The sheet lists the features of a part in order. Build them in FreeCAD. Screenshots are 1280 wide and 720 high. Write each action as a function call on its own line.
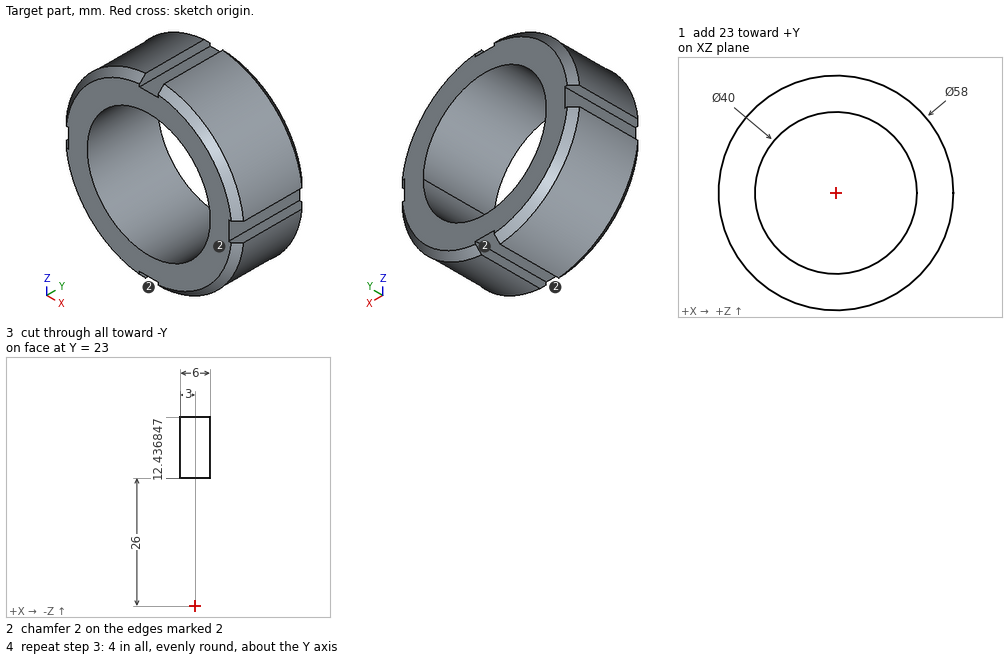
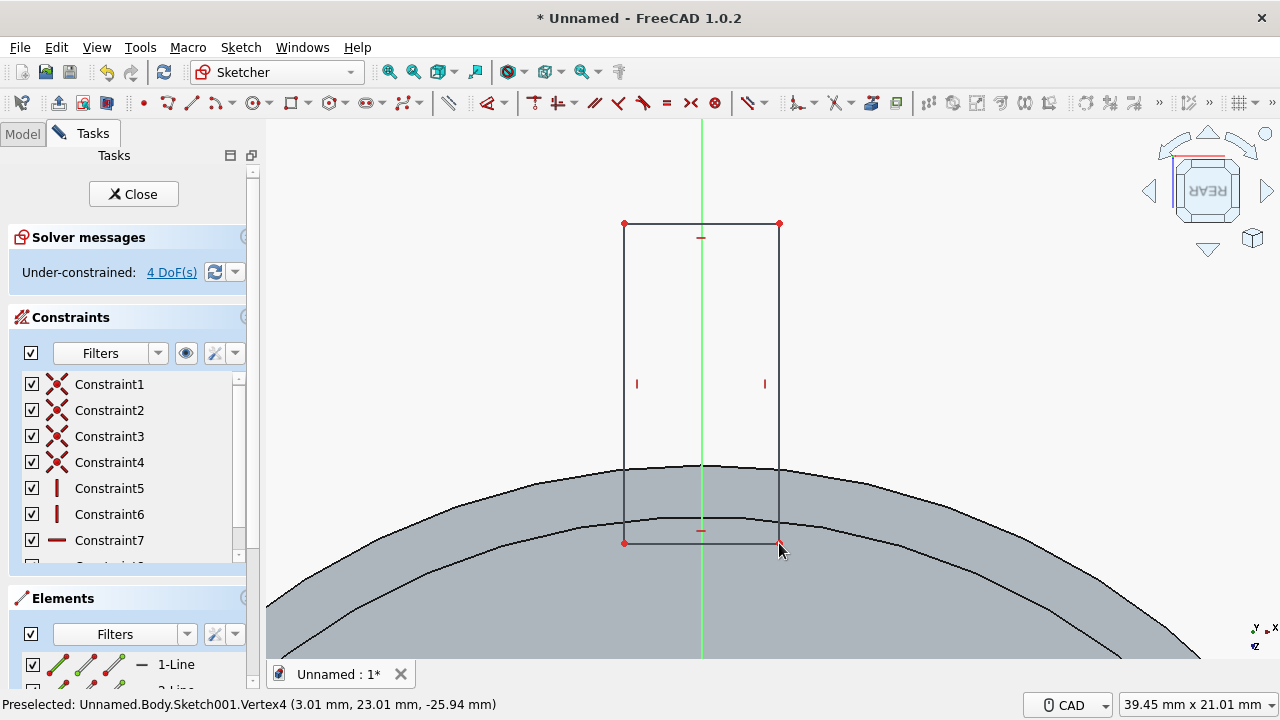
click(488, 104)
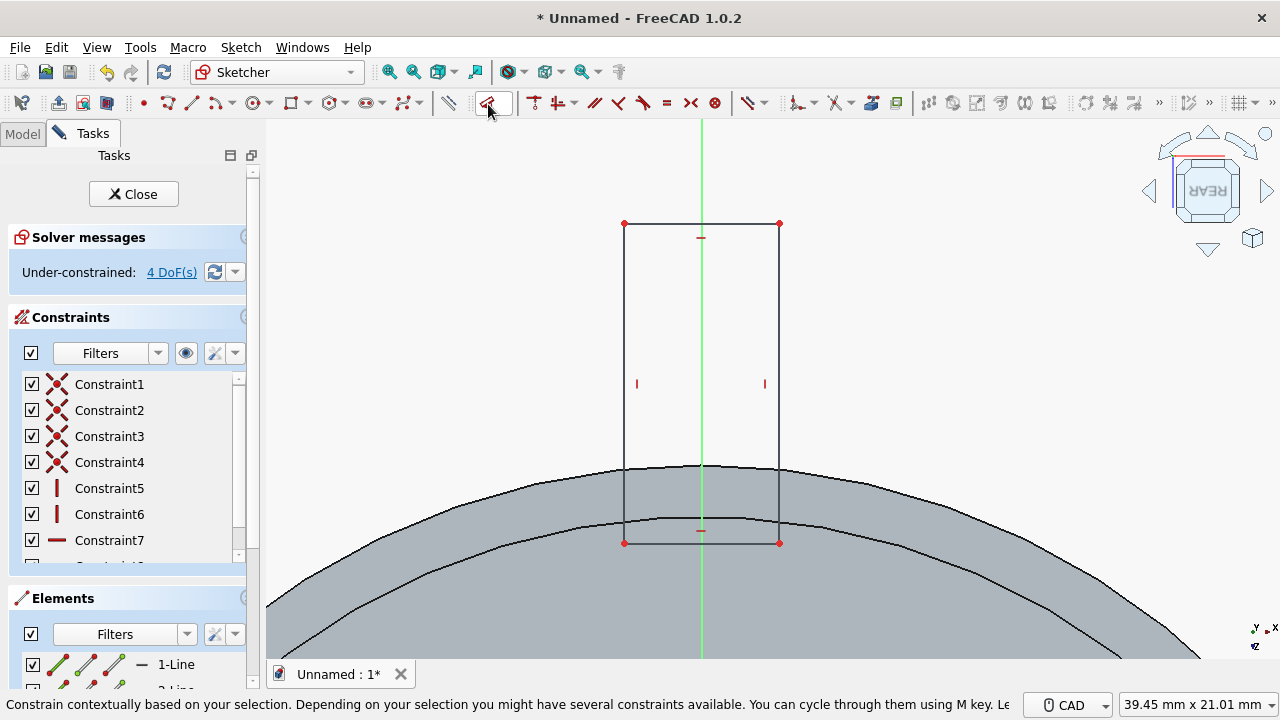
click(671, 544)
click(666, 578)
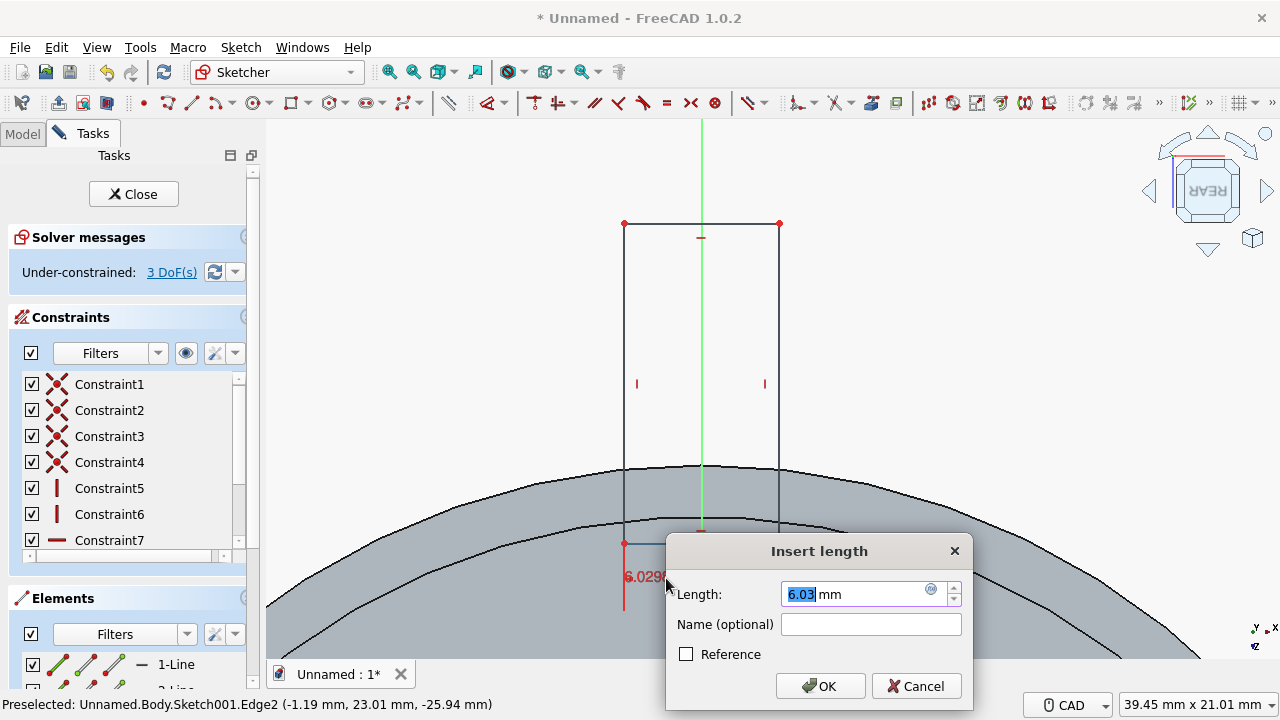
text(6)
key(Return)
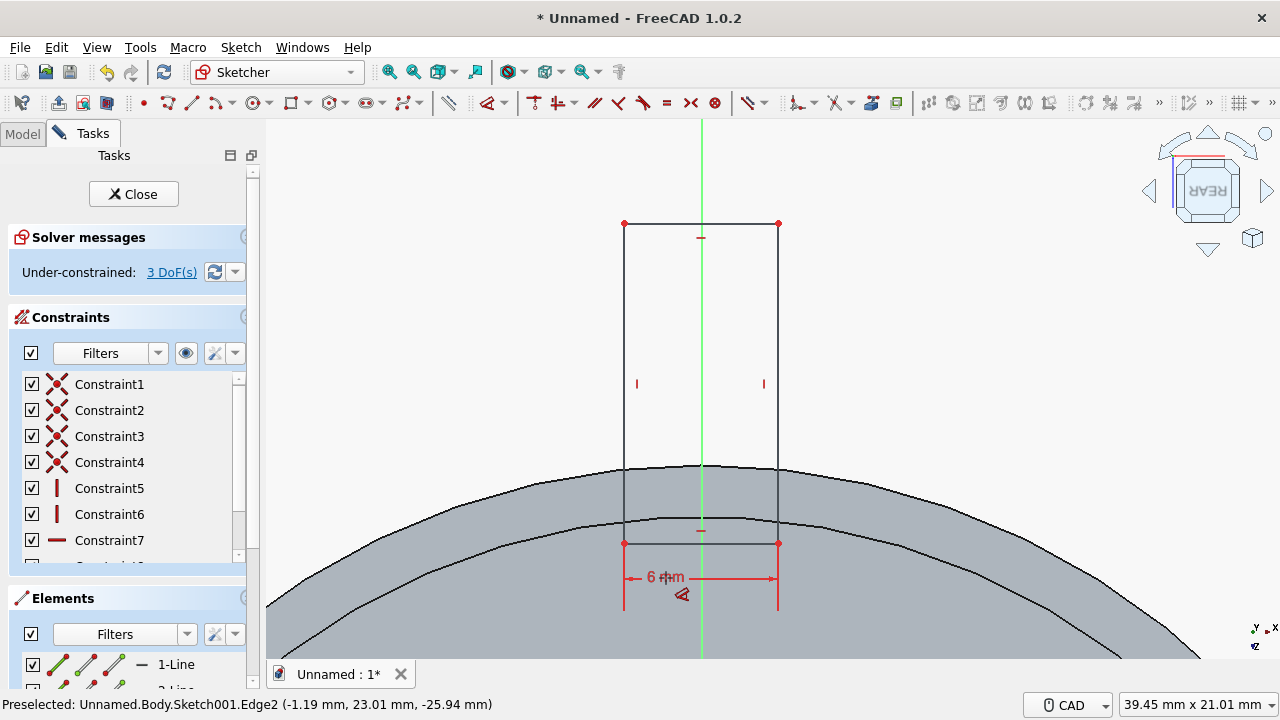
click(624, 224)
click(663, 190)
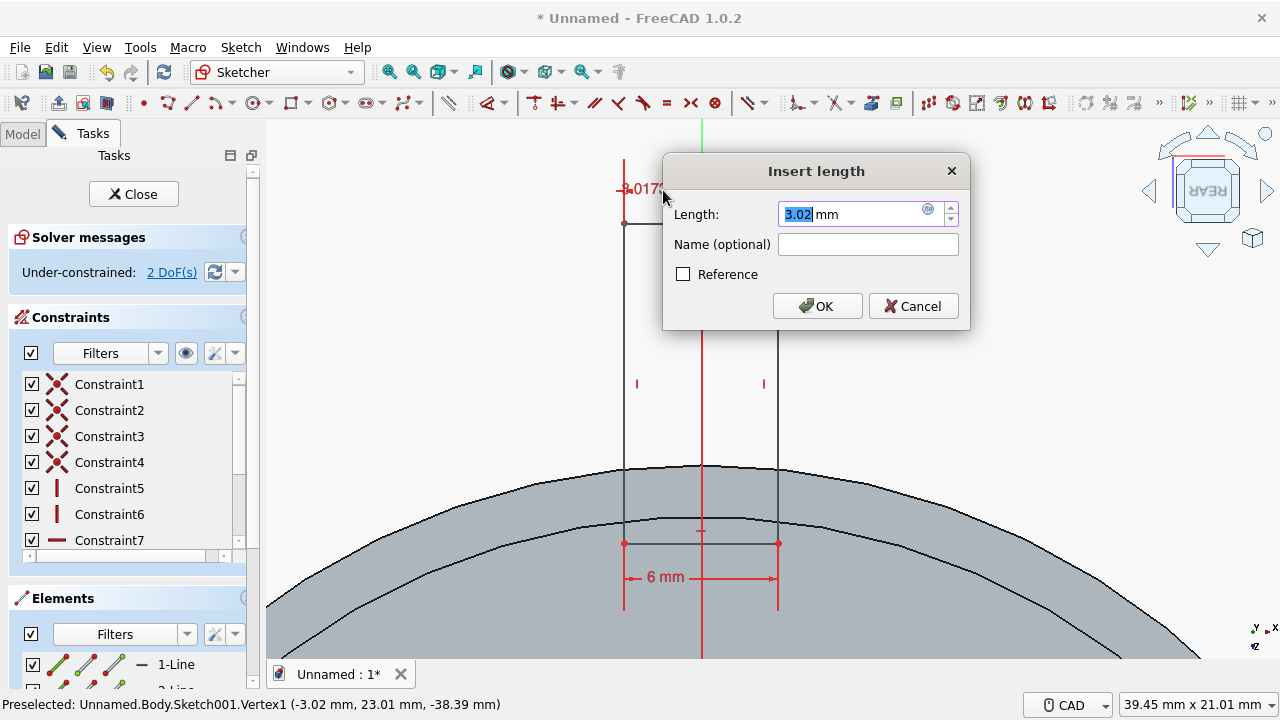
text(3)
key(Return)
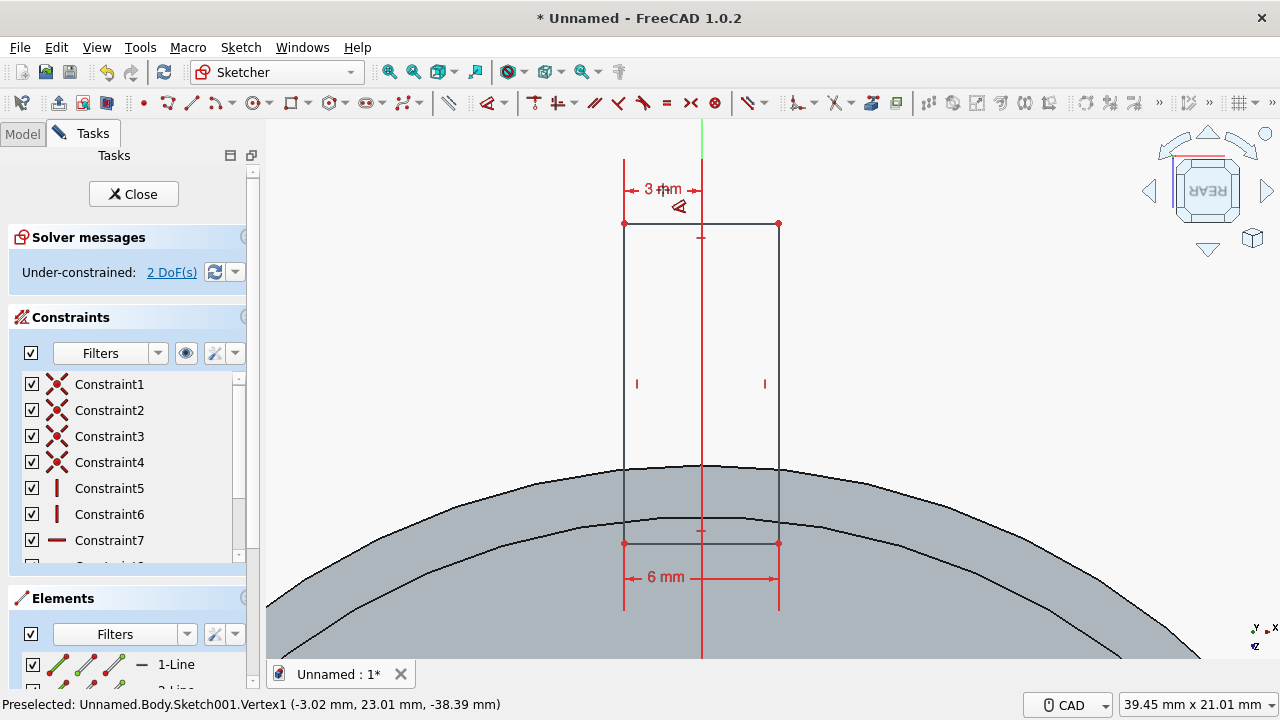
click(624, 544)
click(590, 588)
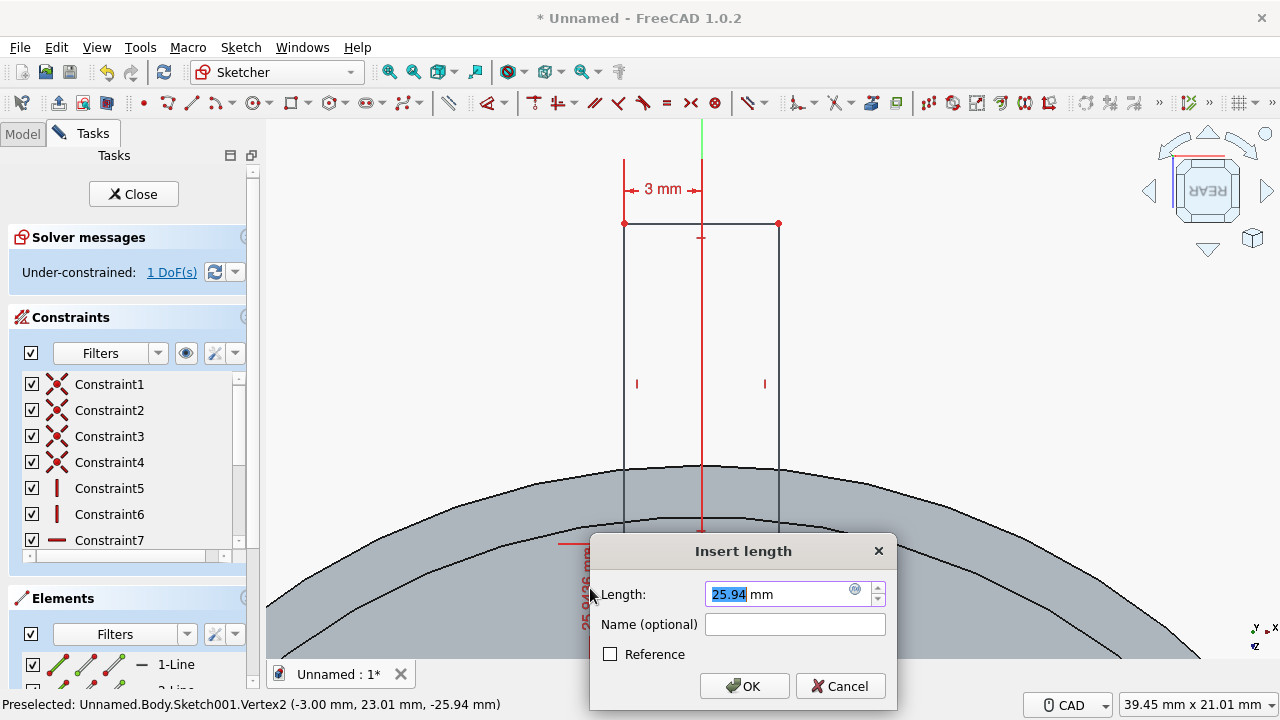
text(26)
key(Return)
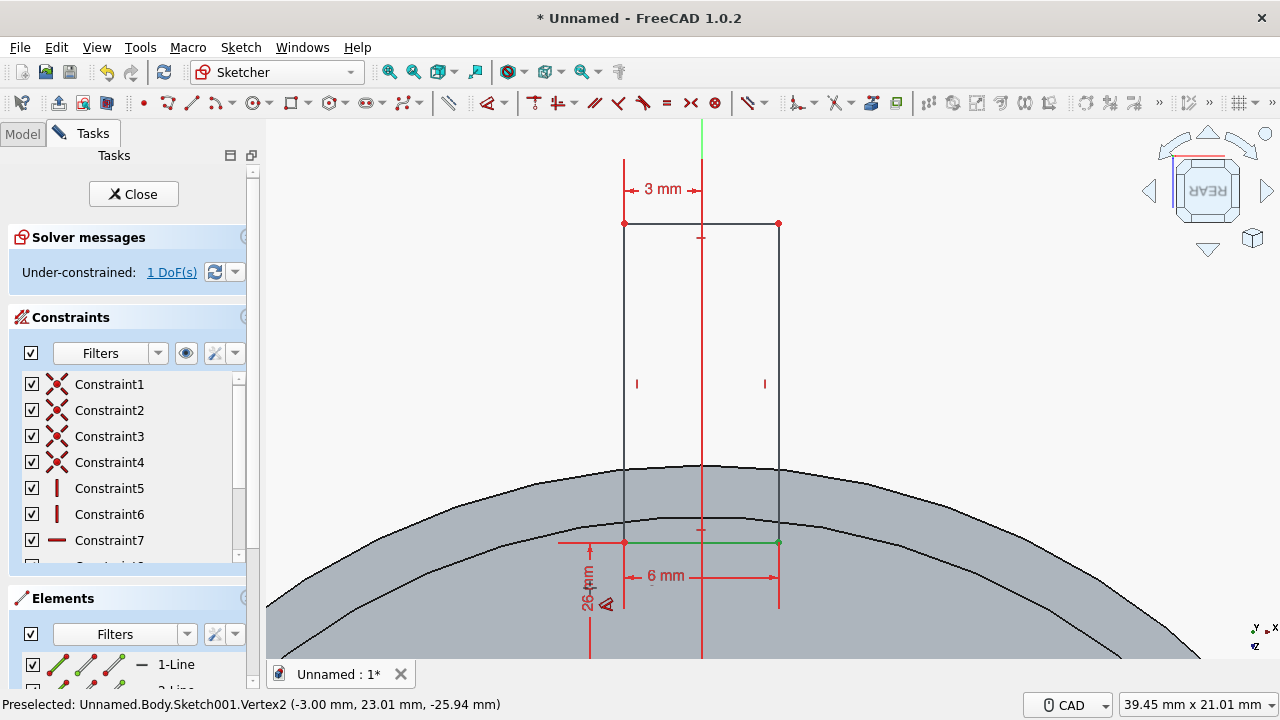
click(624, 320)
click(590, 383)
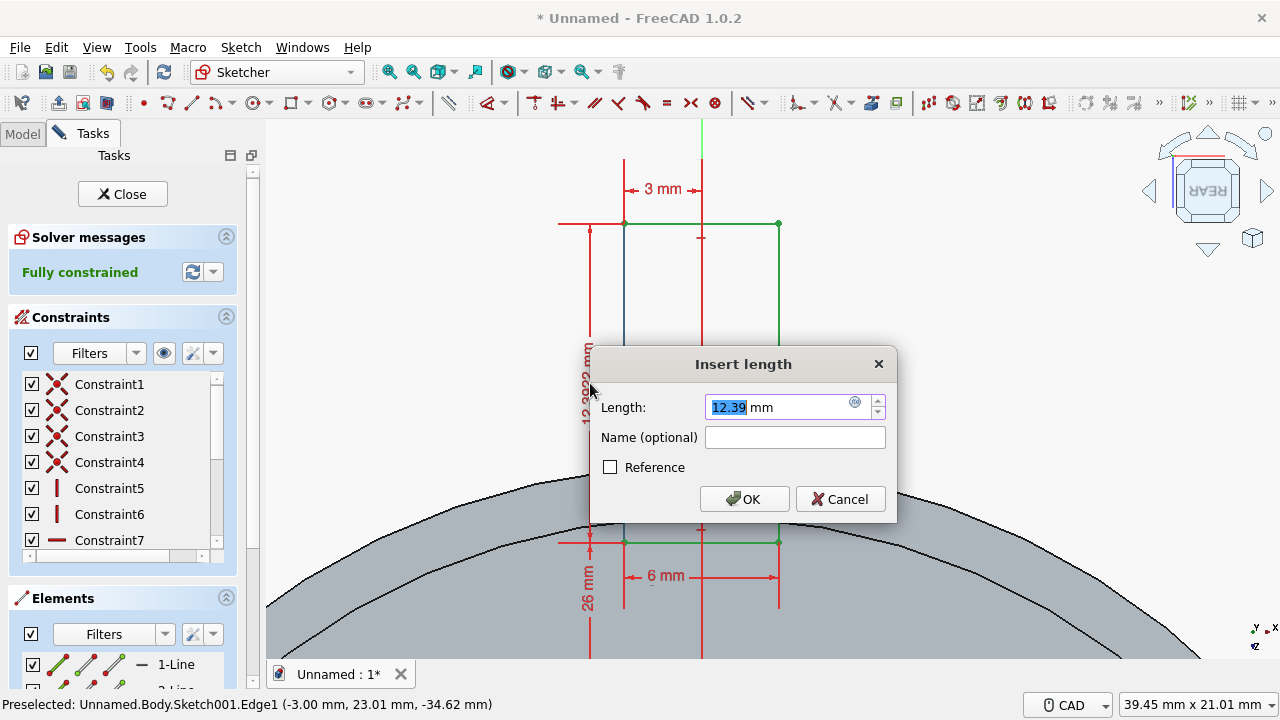
text(12.436847)
key(Return)
key(Escape)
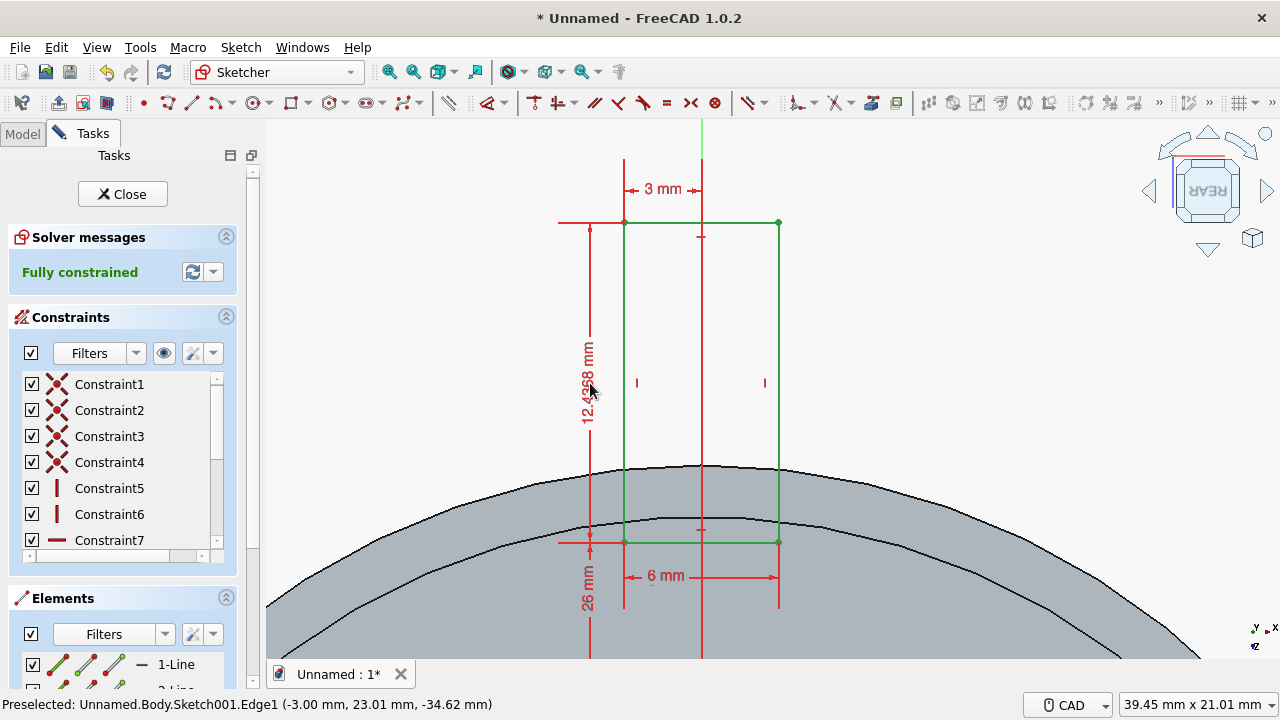
click(123, 194)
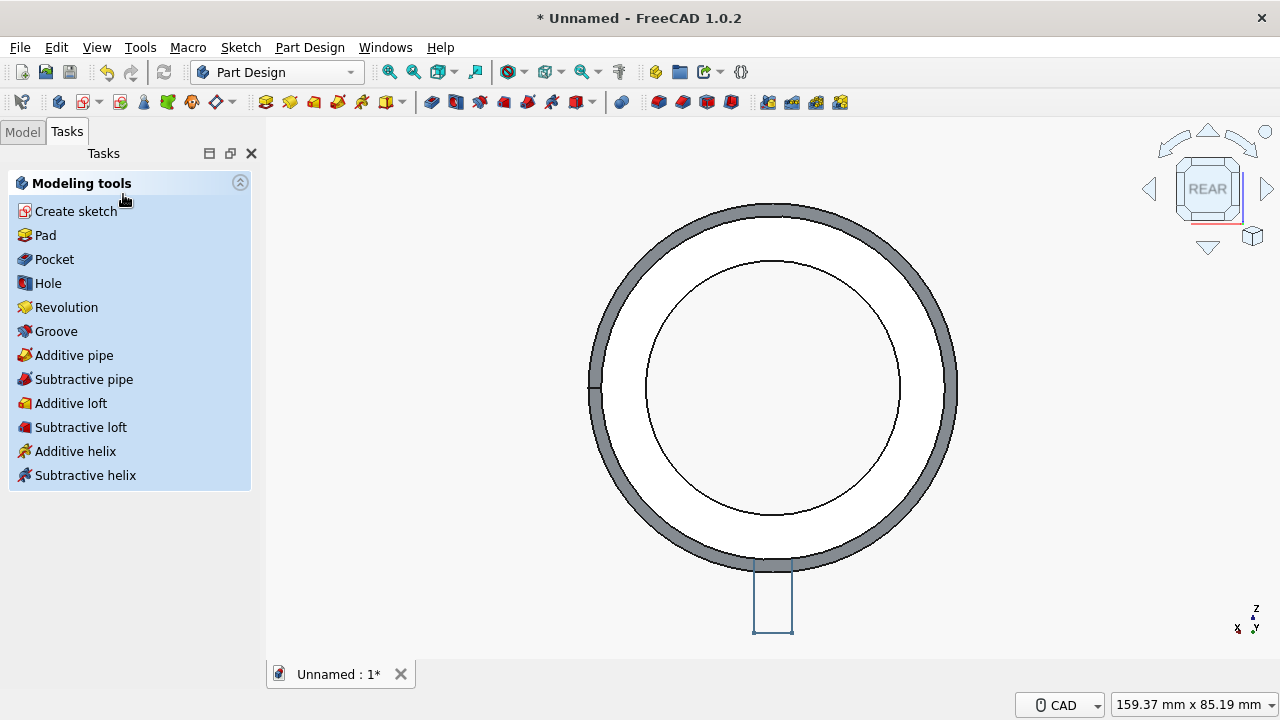
click(432, 102)